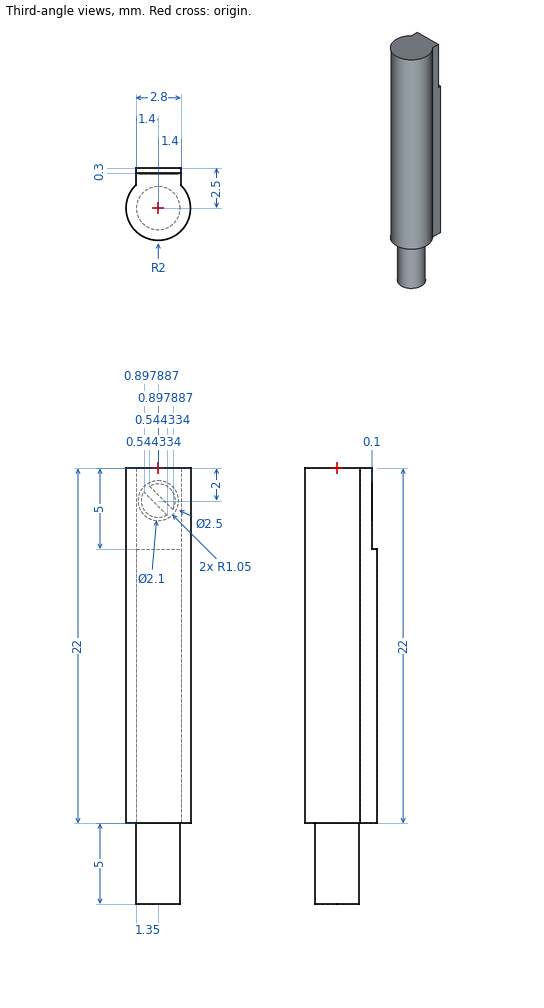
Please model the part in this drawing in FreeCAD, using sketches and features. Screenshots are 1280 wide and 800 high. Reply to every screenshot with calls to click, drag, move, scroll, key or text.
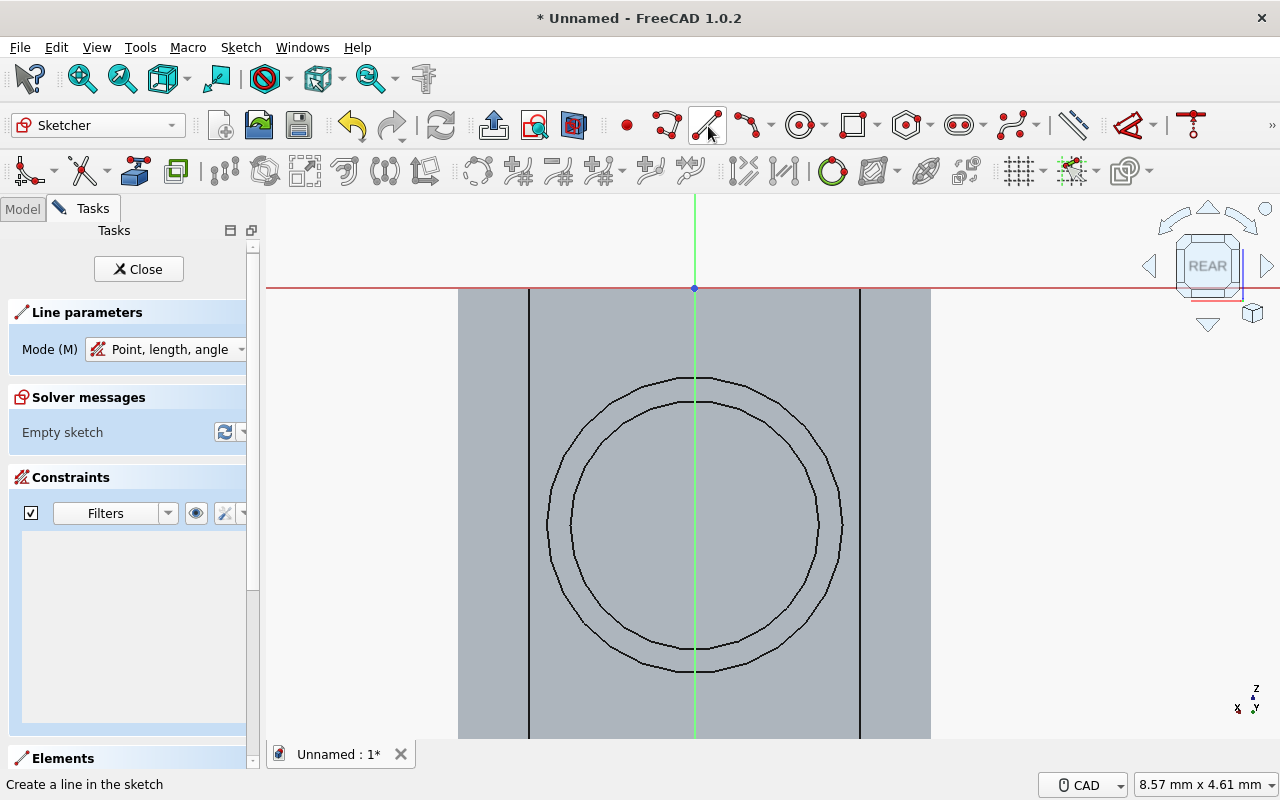
click(759, 419)
click(588, 590)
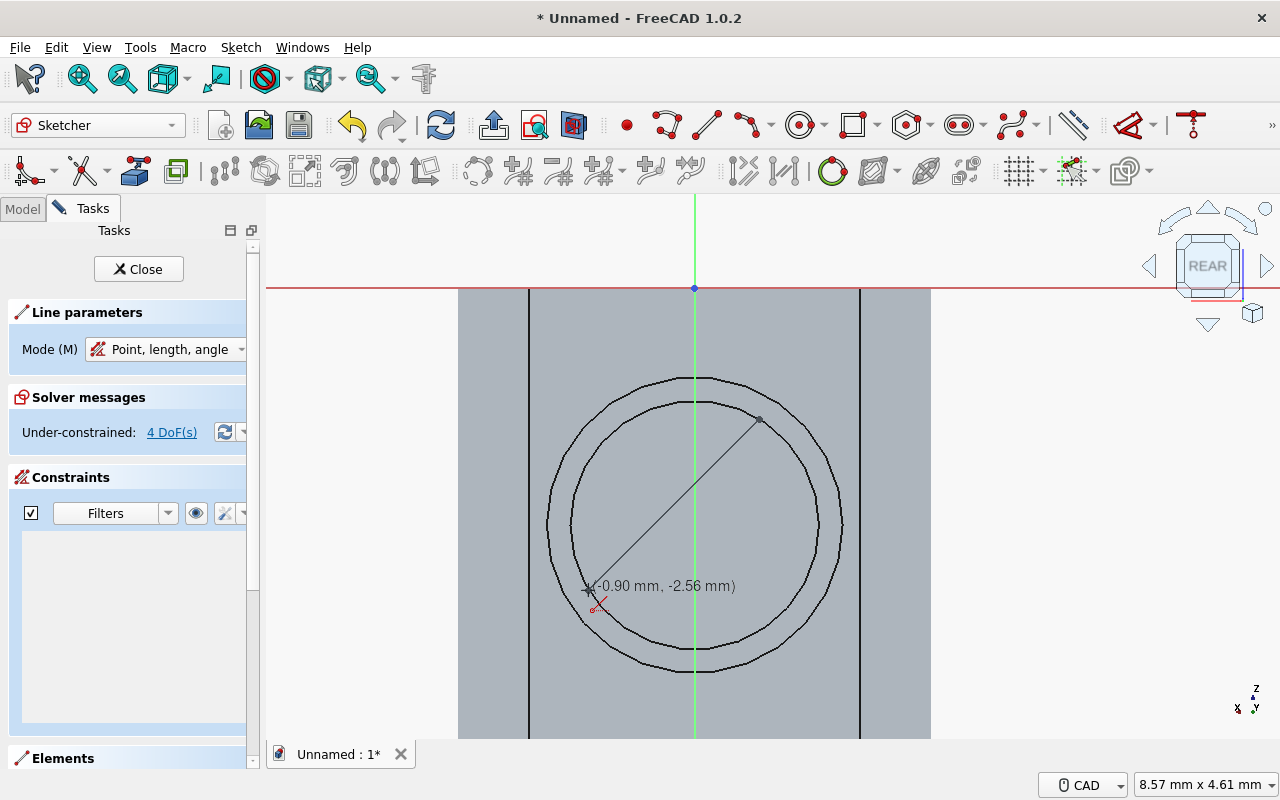
click(630, 631)
click(801, 461)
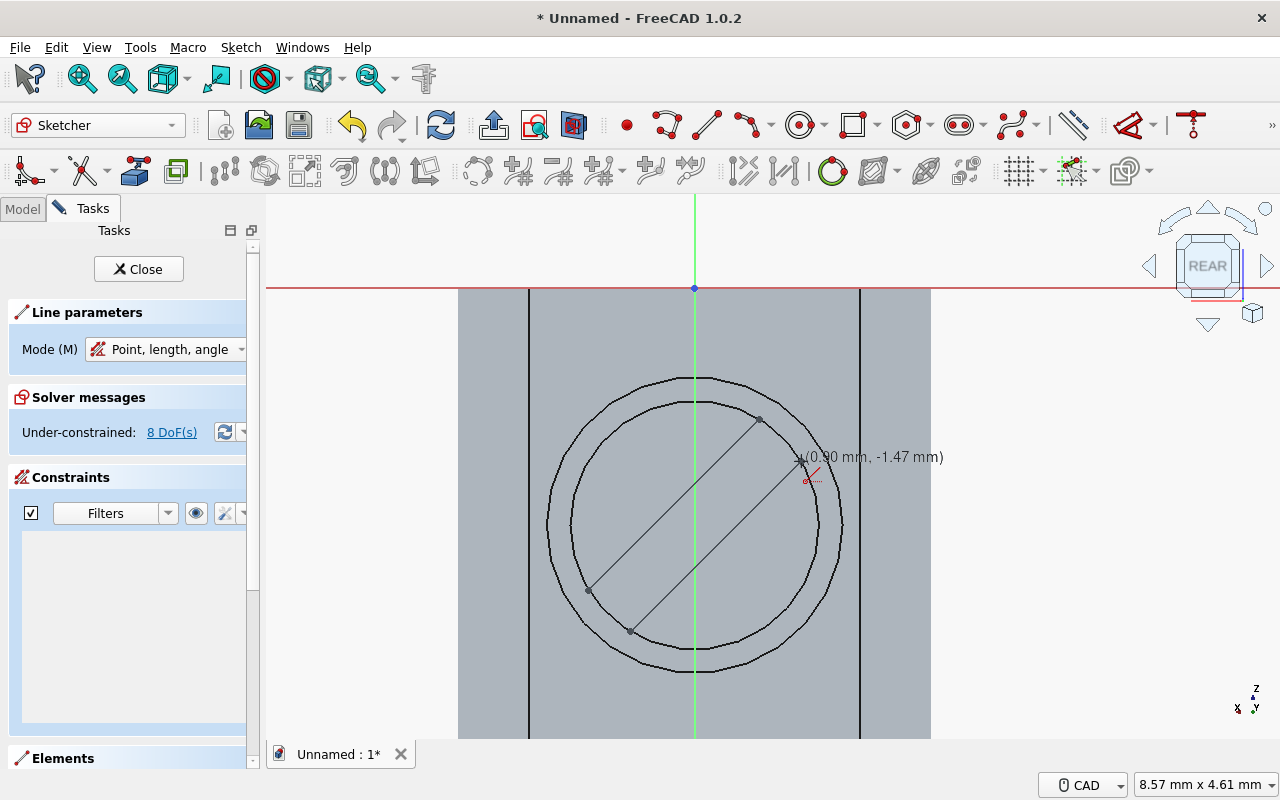
click(748, 126)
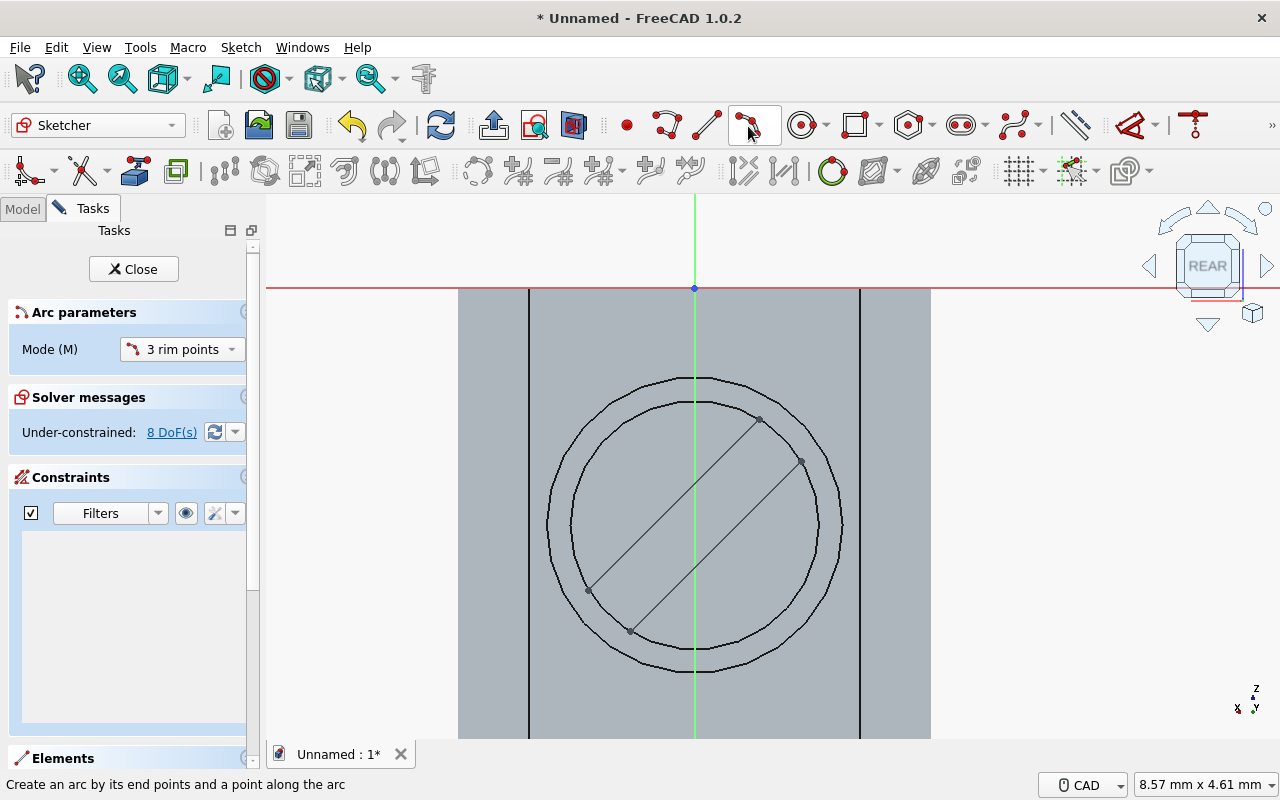
click(588, 591)
click(630, 632)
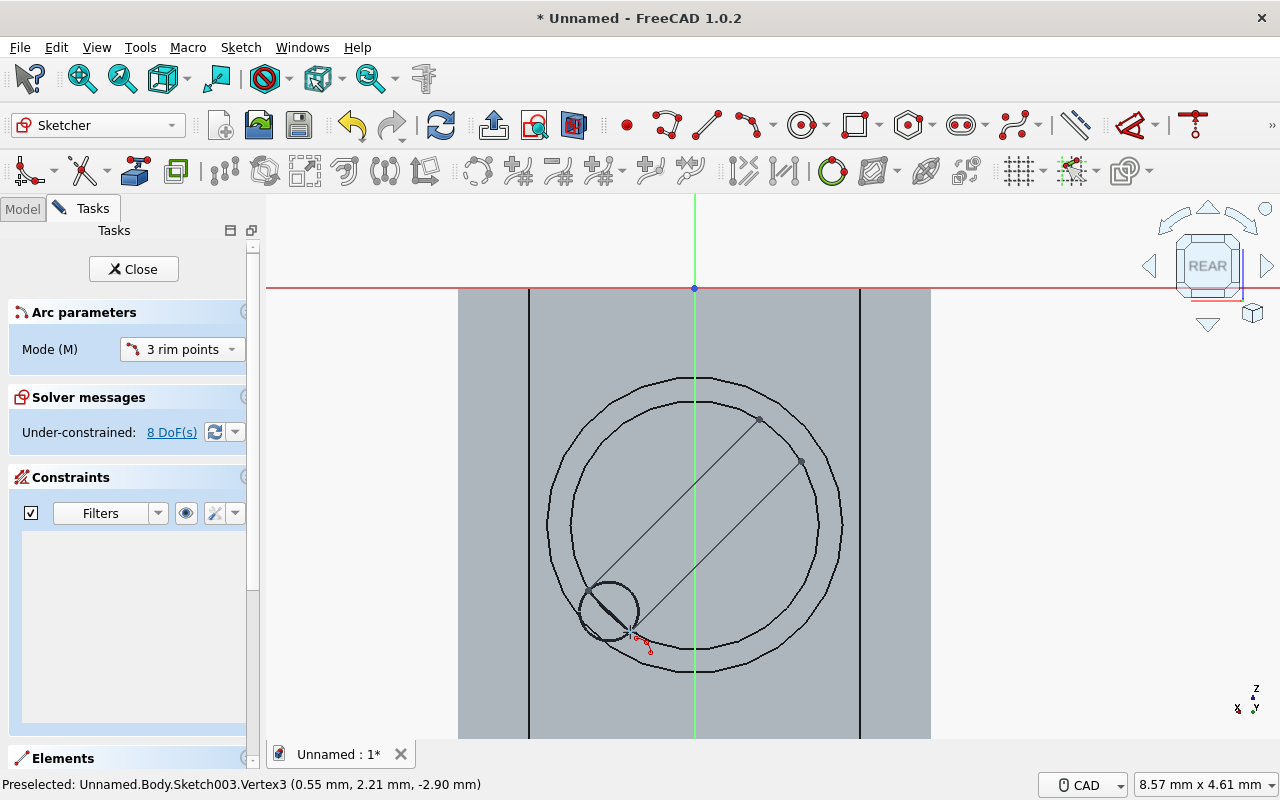
scroll(607, 613, up, 8)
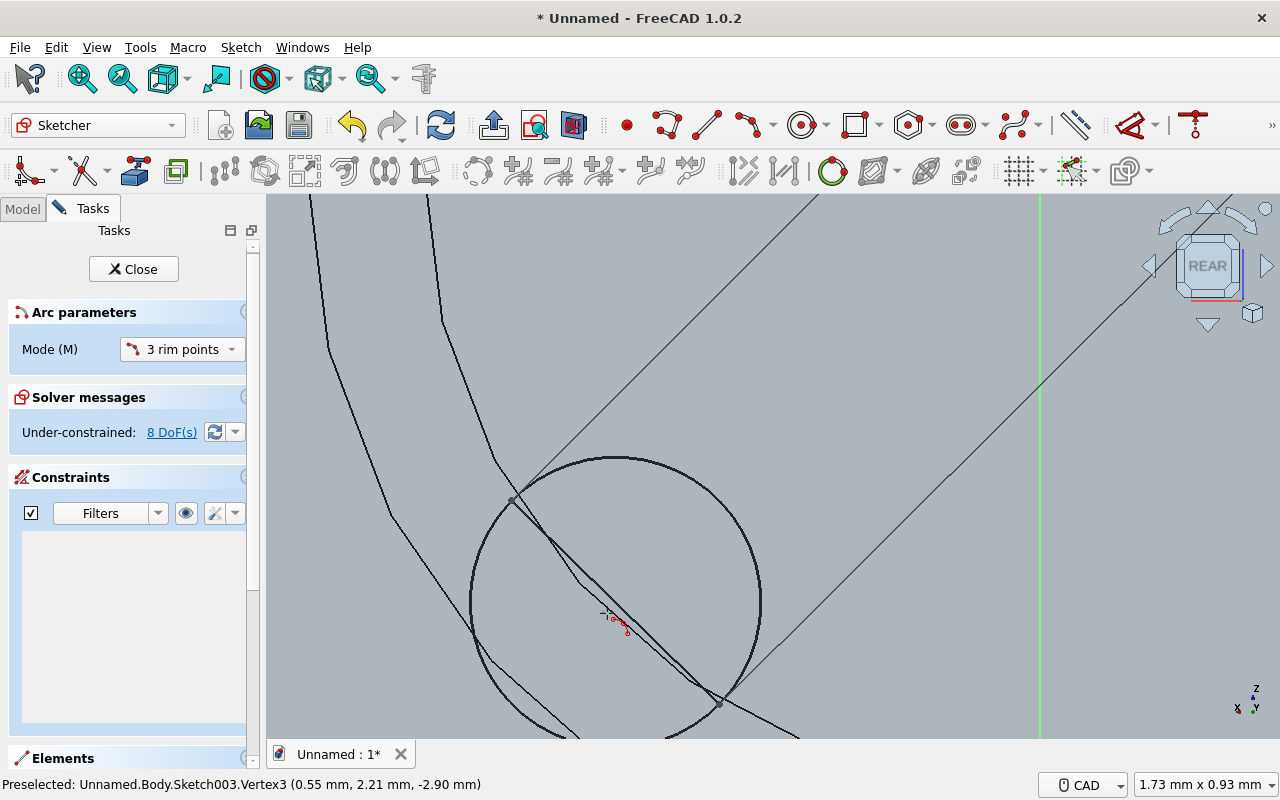
click(605, 610)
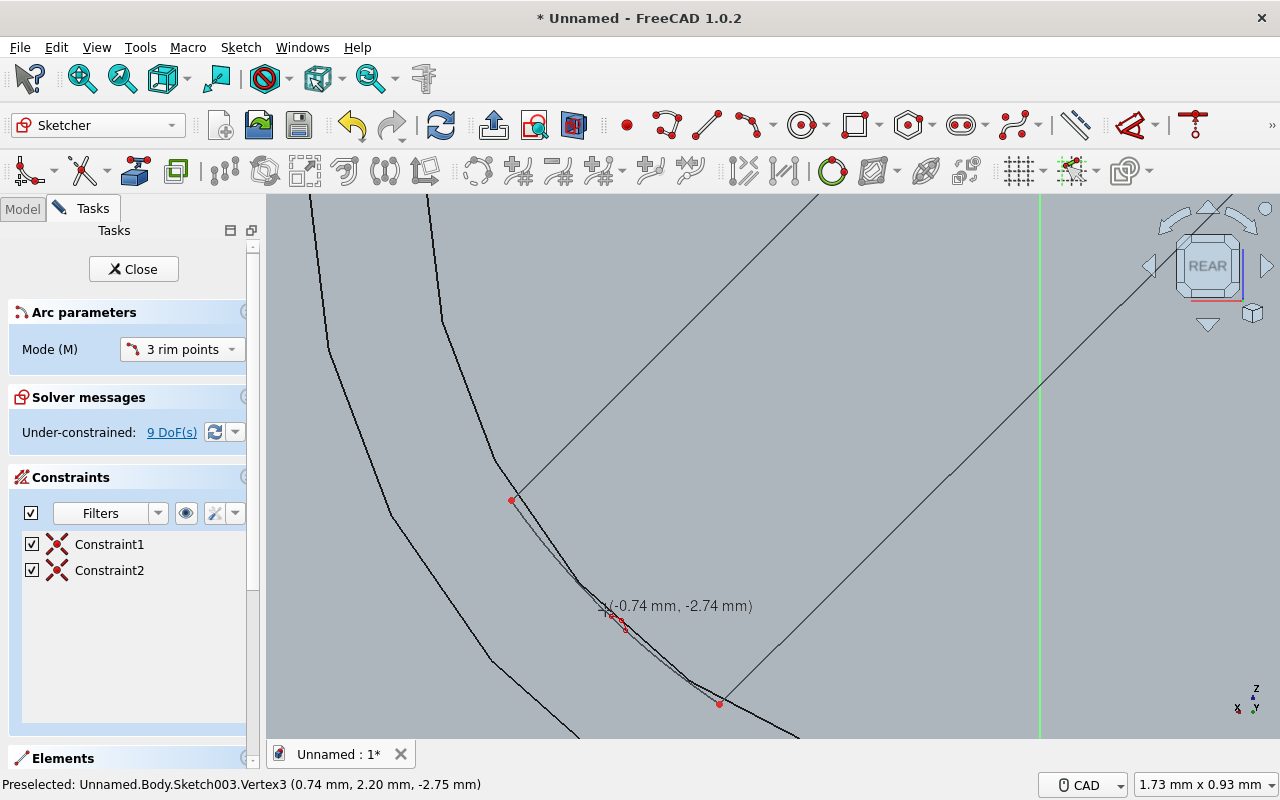
scroll(620, 622, down, 8)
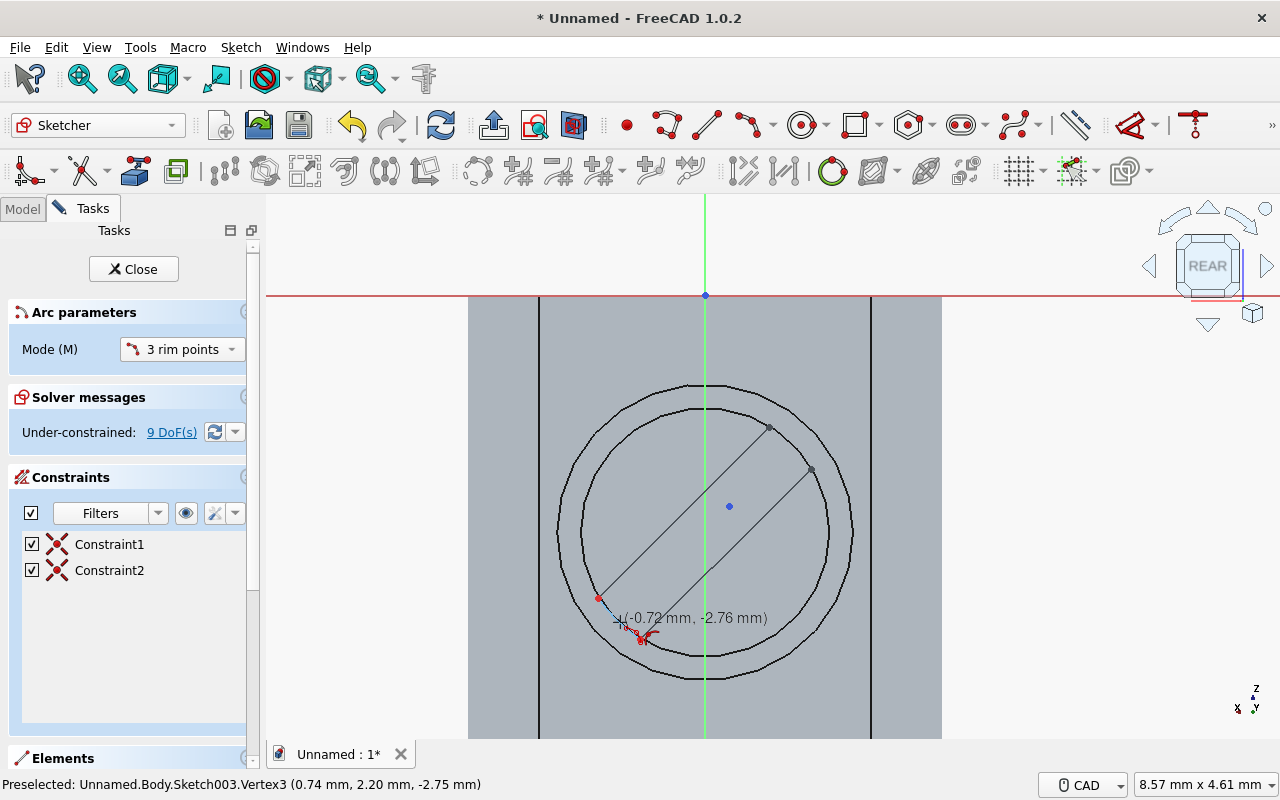
click(811, 469)
click(769, 427)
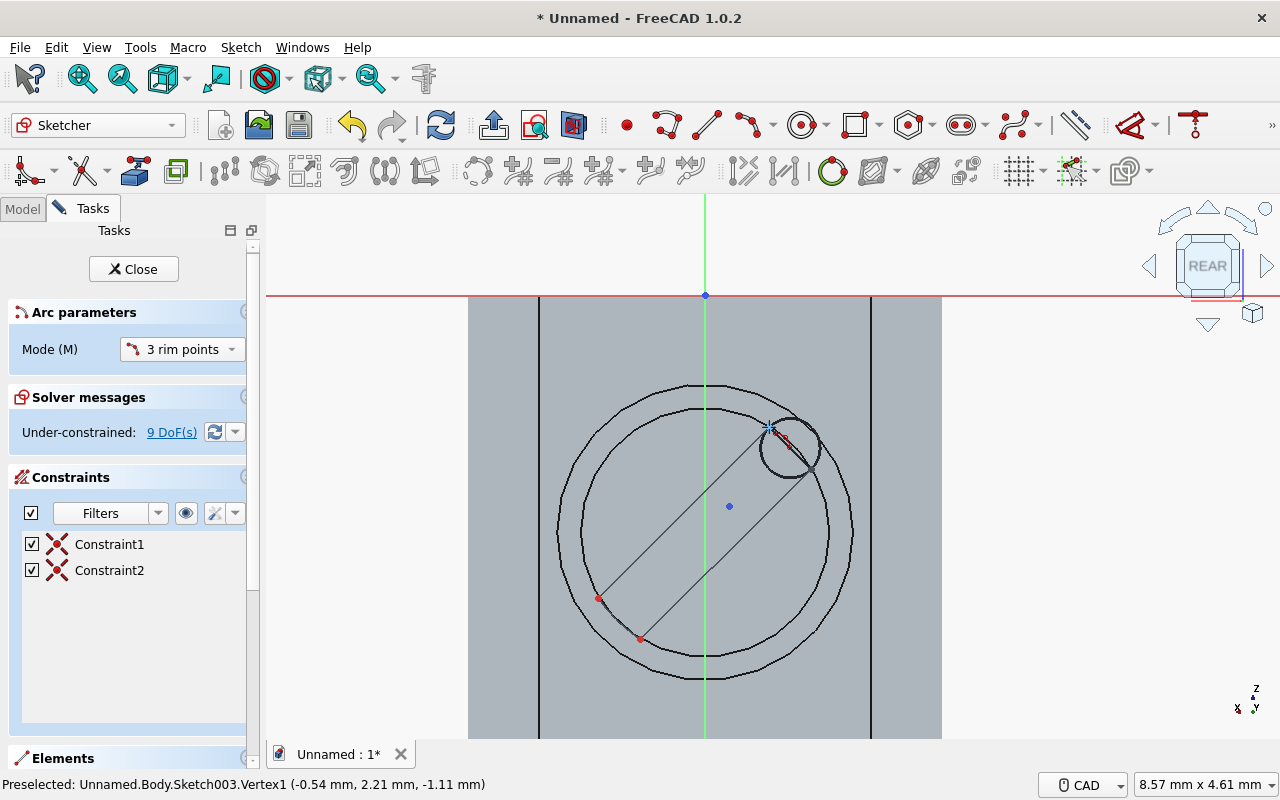
scroll(793, 444, up, 8)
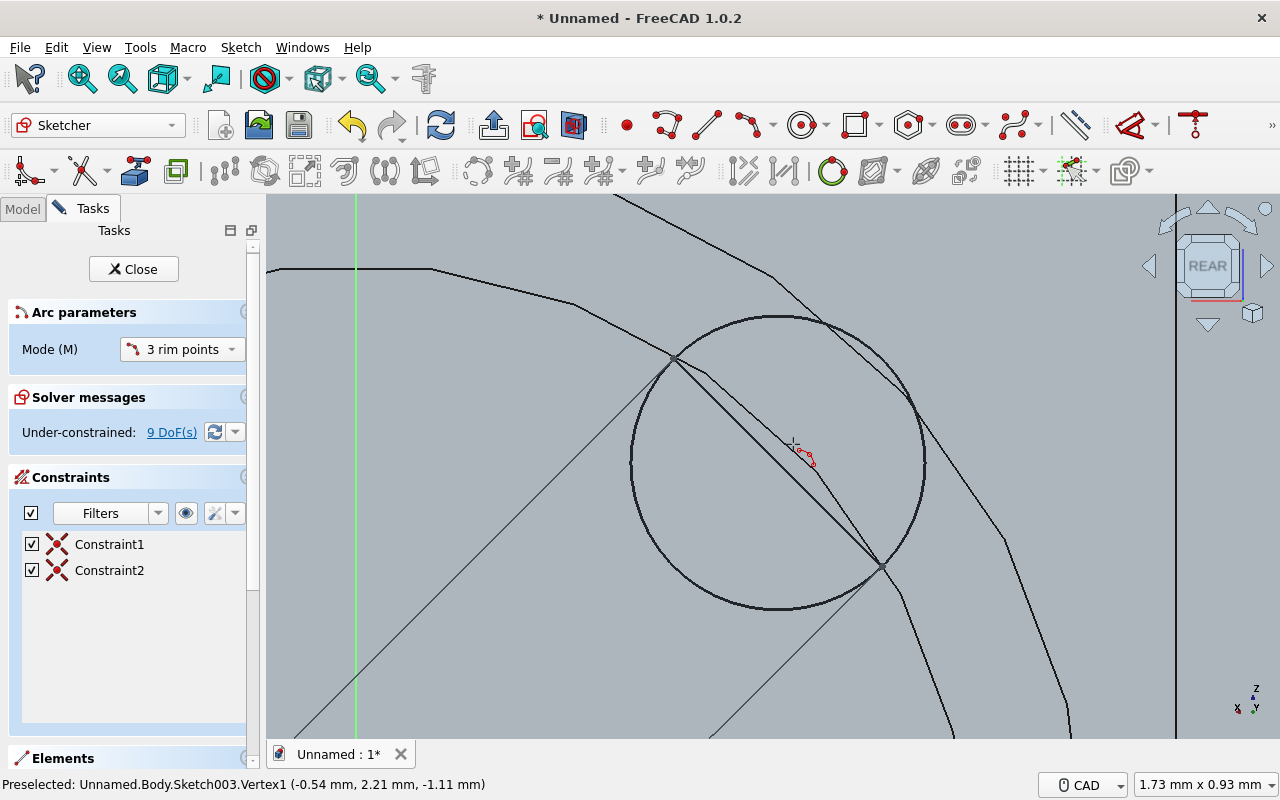
click(791, 445)
key(Escape)